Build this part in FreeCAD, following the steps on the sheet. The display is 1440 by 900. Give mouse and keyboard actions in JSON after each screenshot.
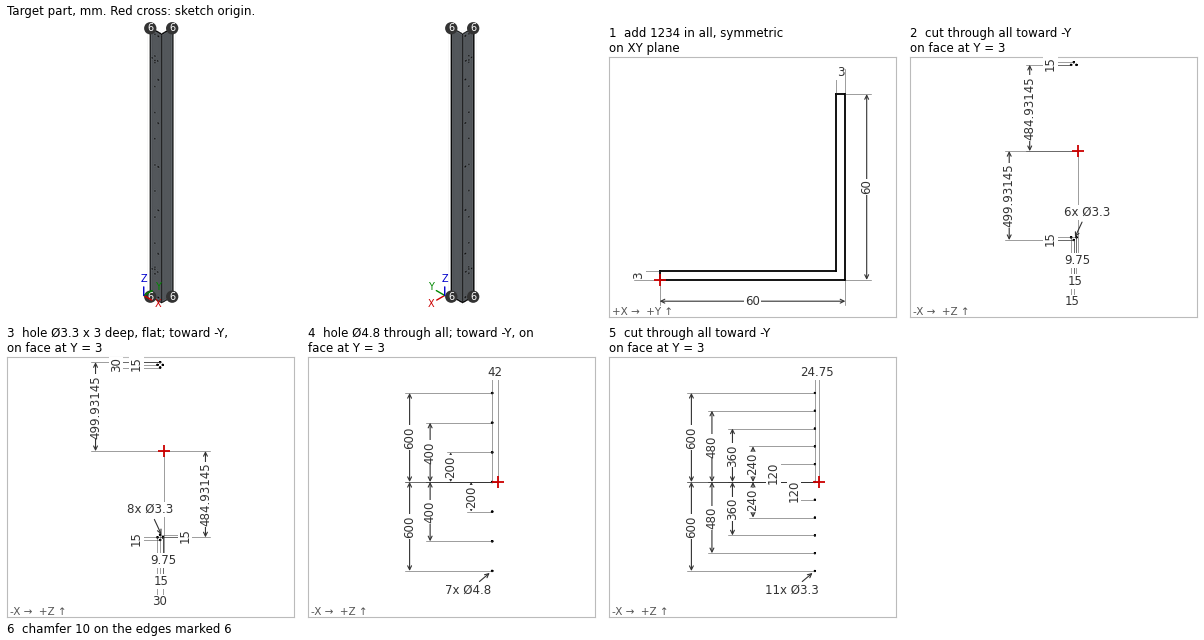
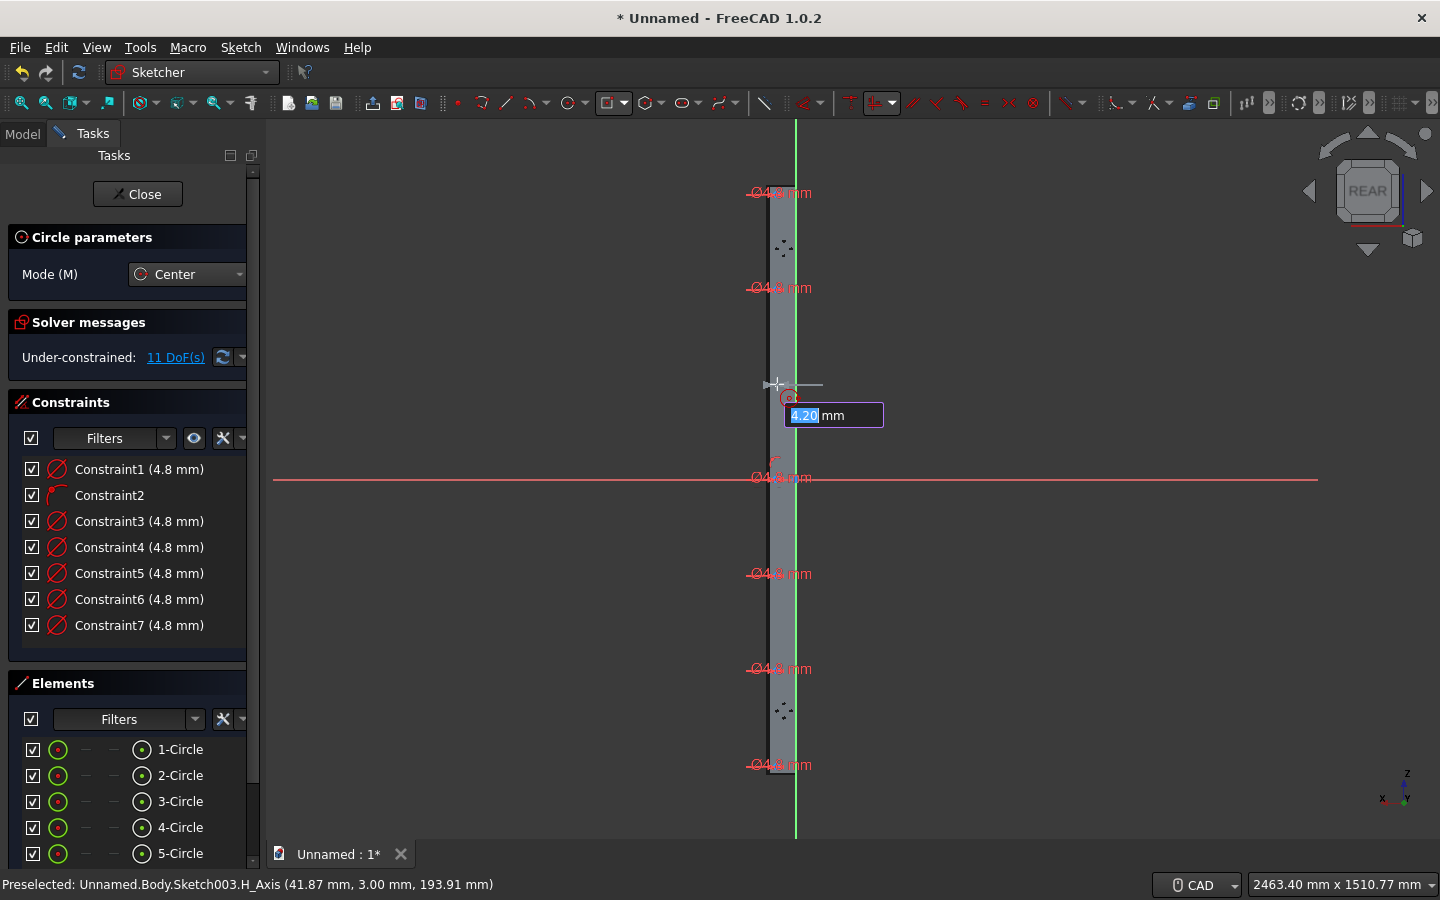
{"action": "type", "text": "4.8"}
{"action": "key", "text": "Return"}
{"action": "key", "text": "Escape"}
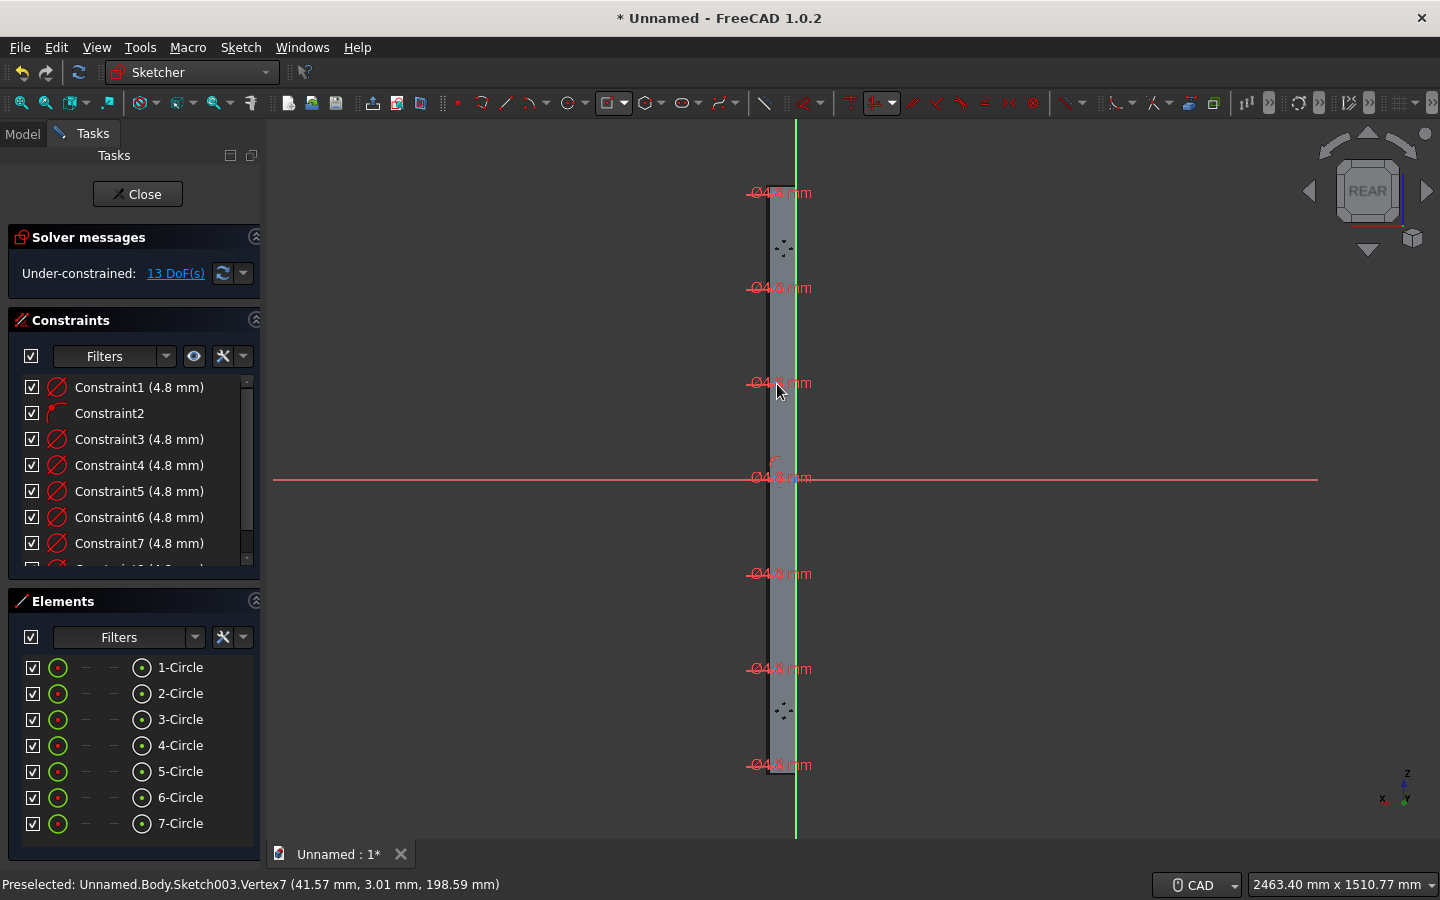
{"action": "left_click", "coordinate": [776, 480]}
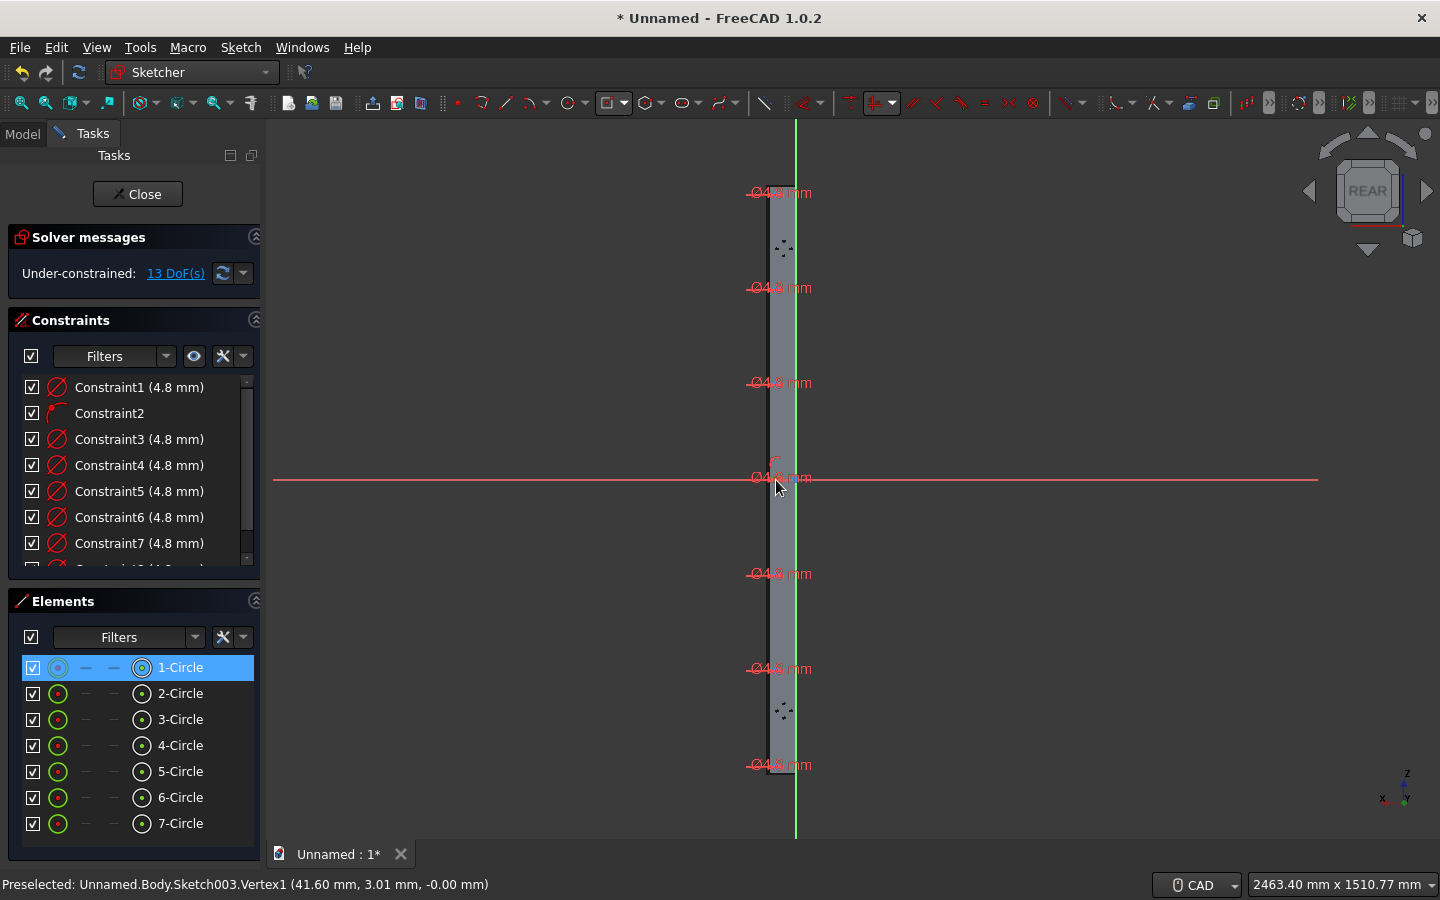
{"action": "left_click", "coordinate": [776, 576]}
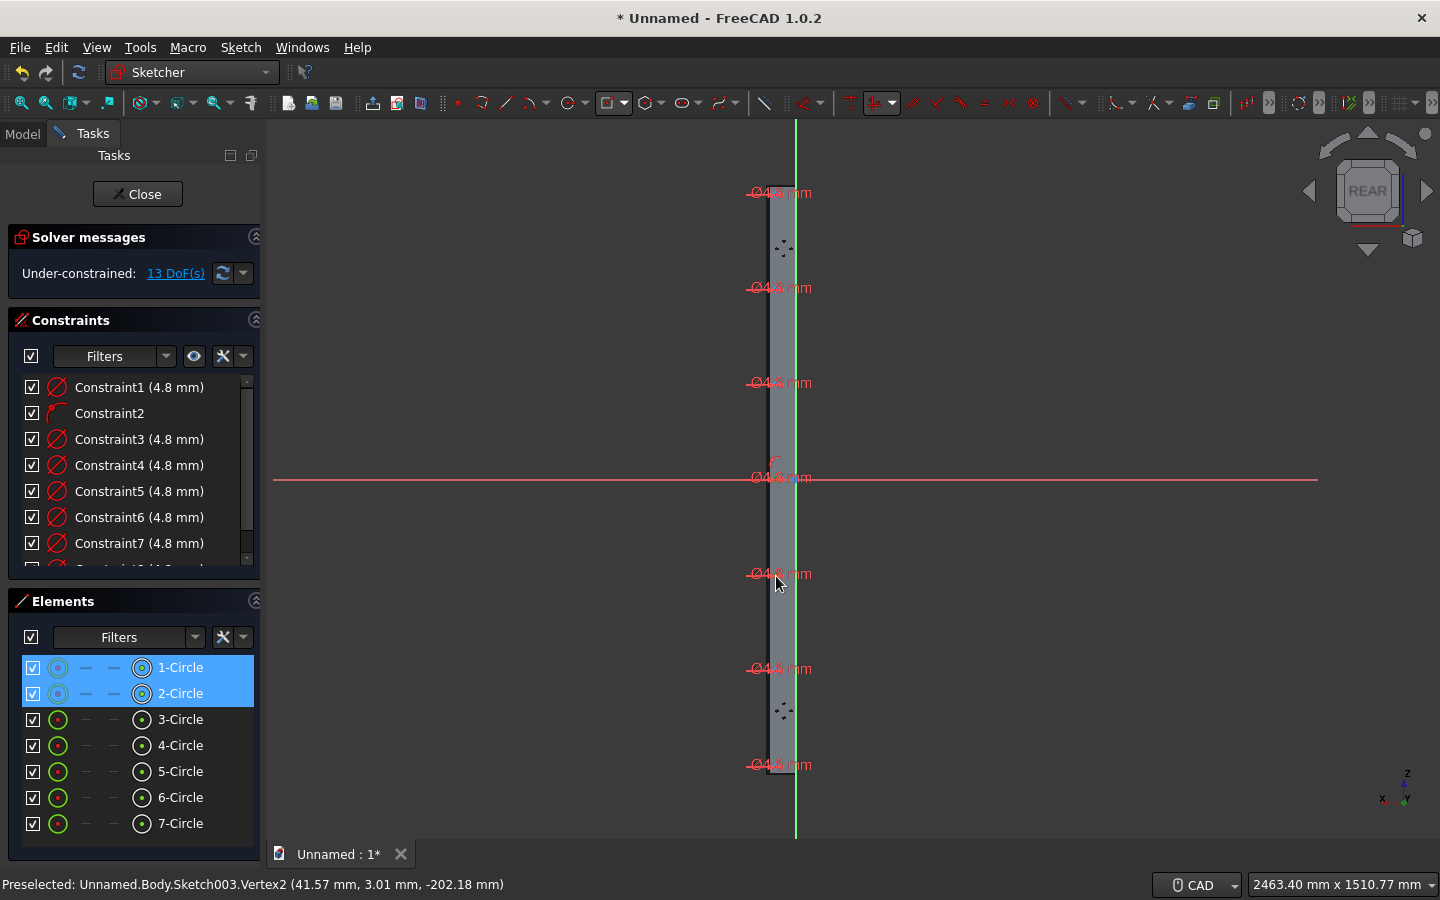
{"action": "left_click", "coordinate": [894, 104]}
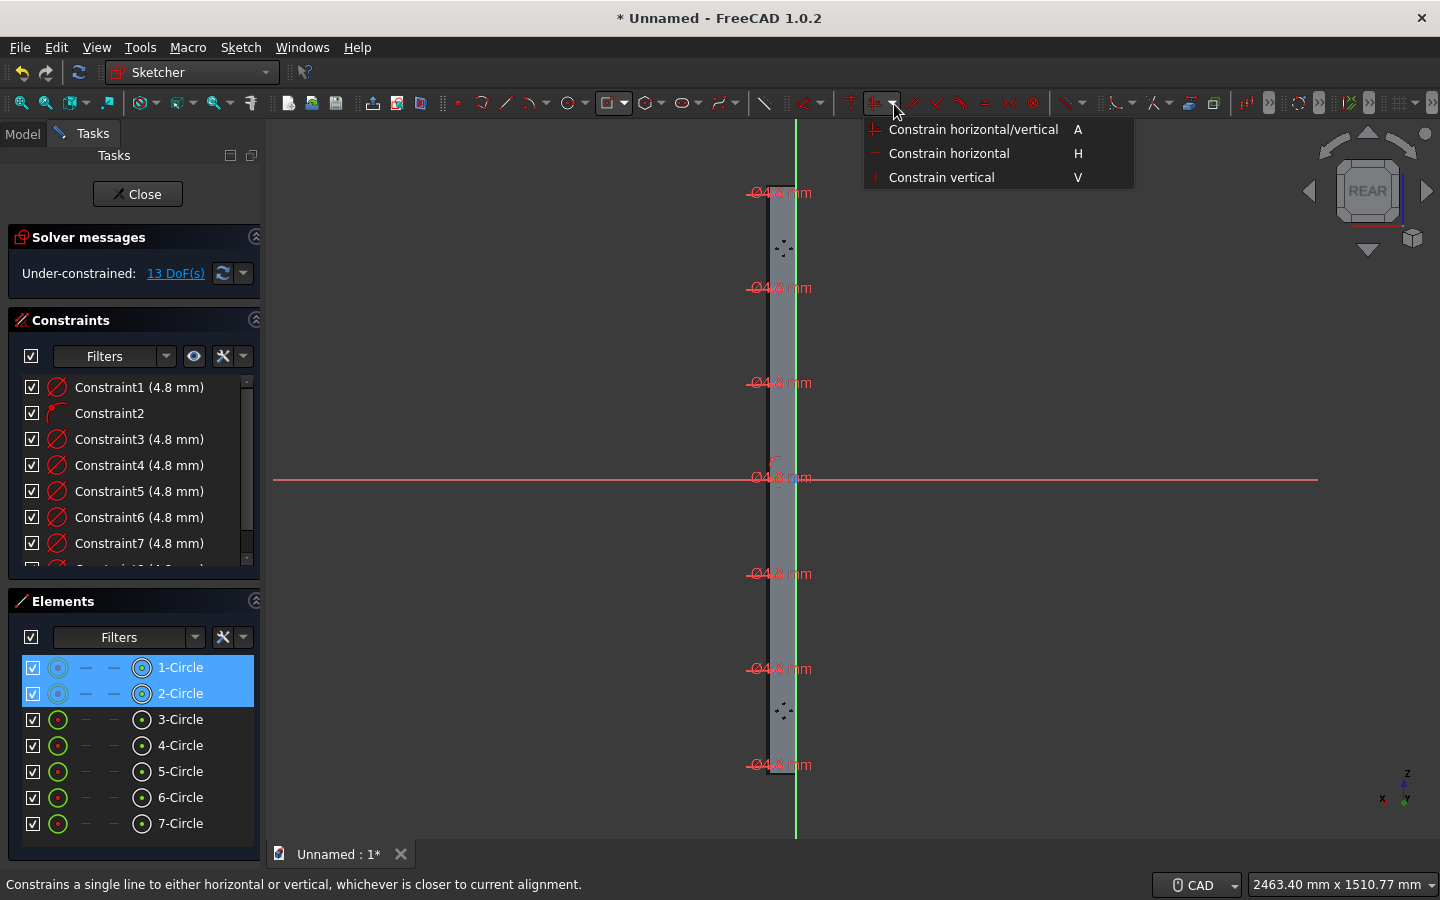
{"action": "left_click", "coordinate": [999, 177]}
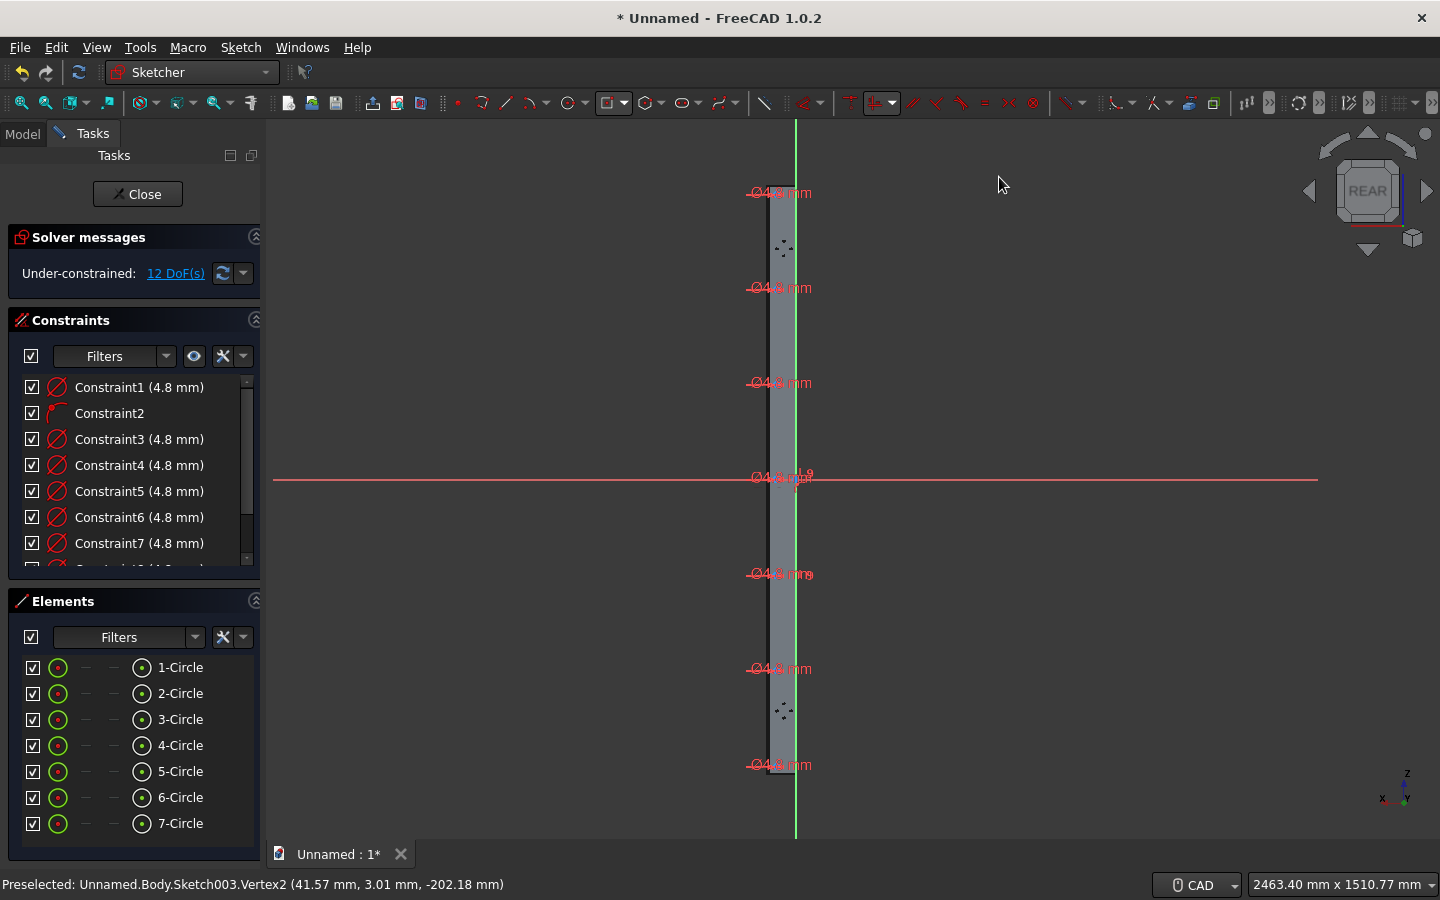
{"action": "left_click", "coordinate": [776, 576]}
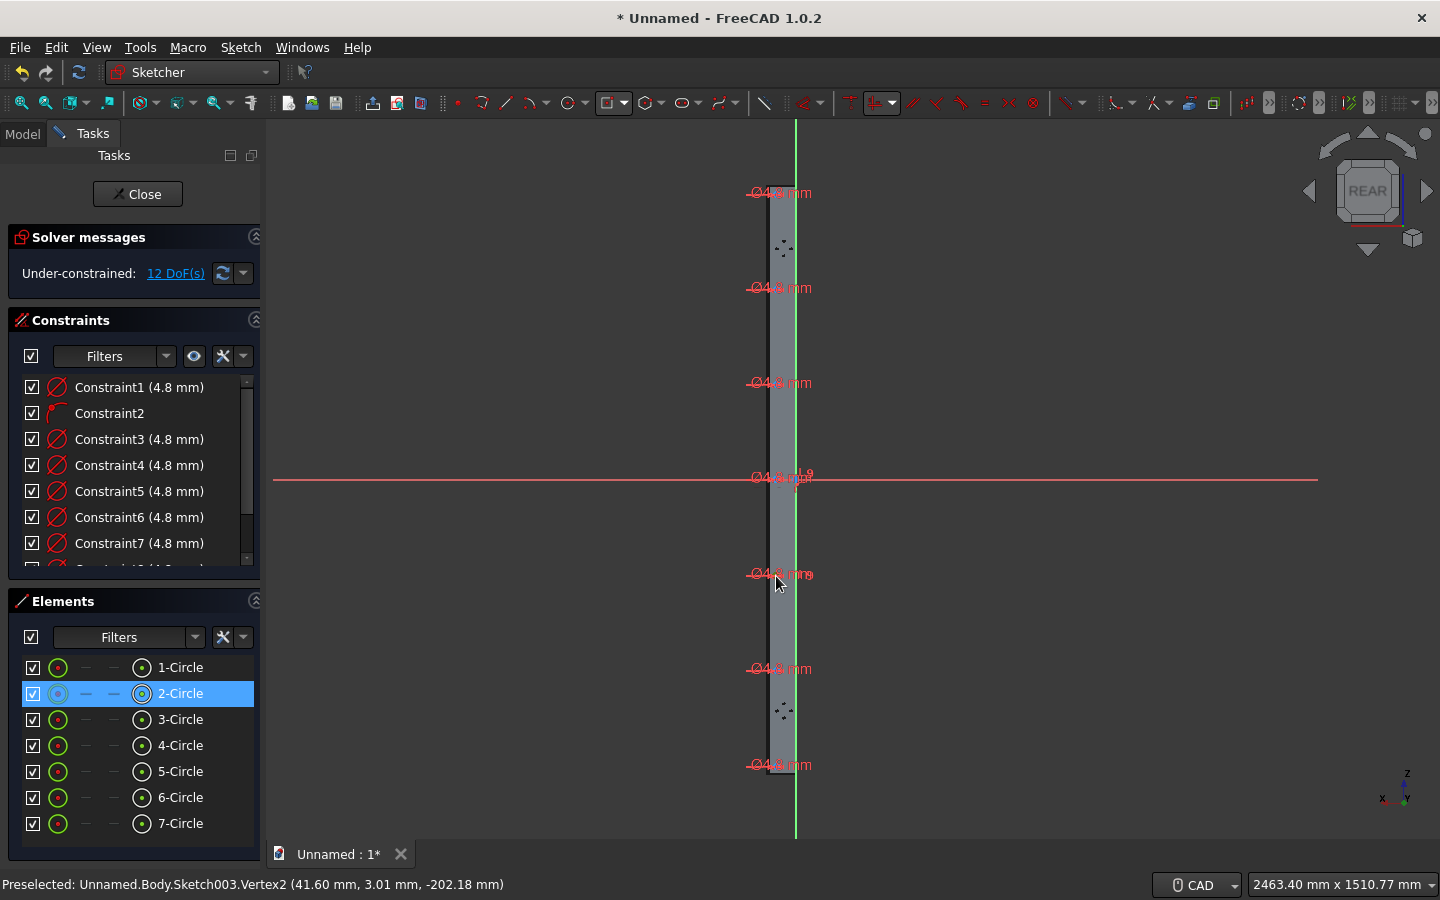
{"action": "left_click", "coordinate": [776, 671]}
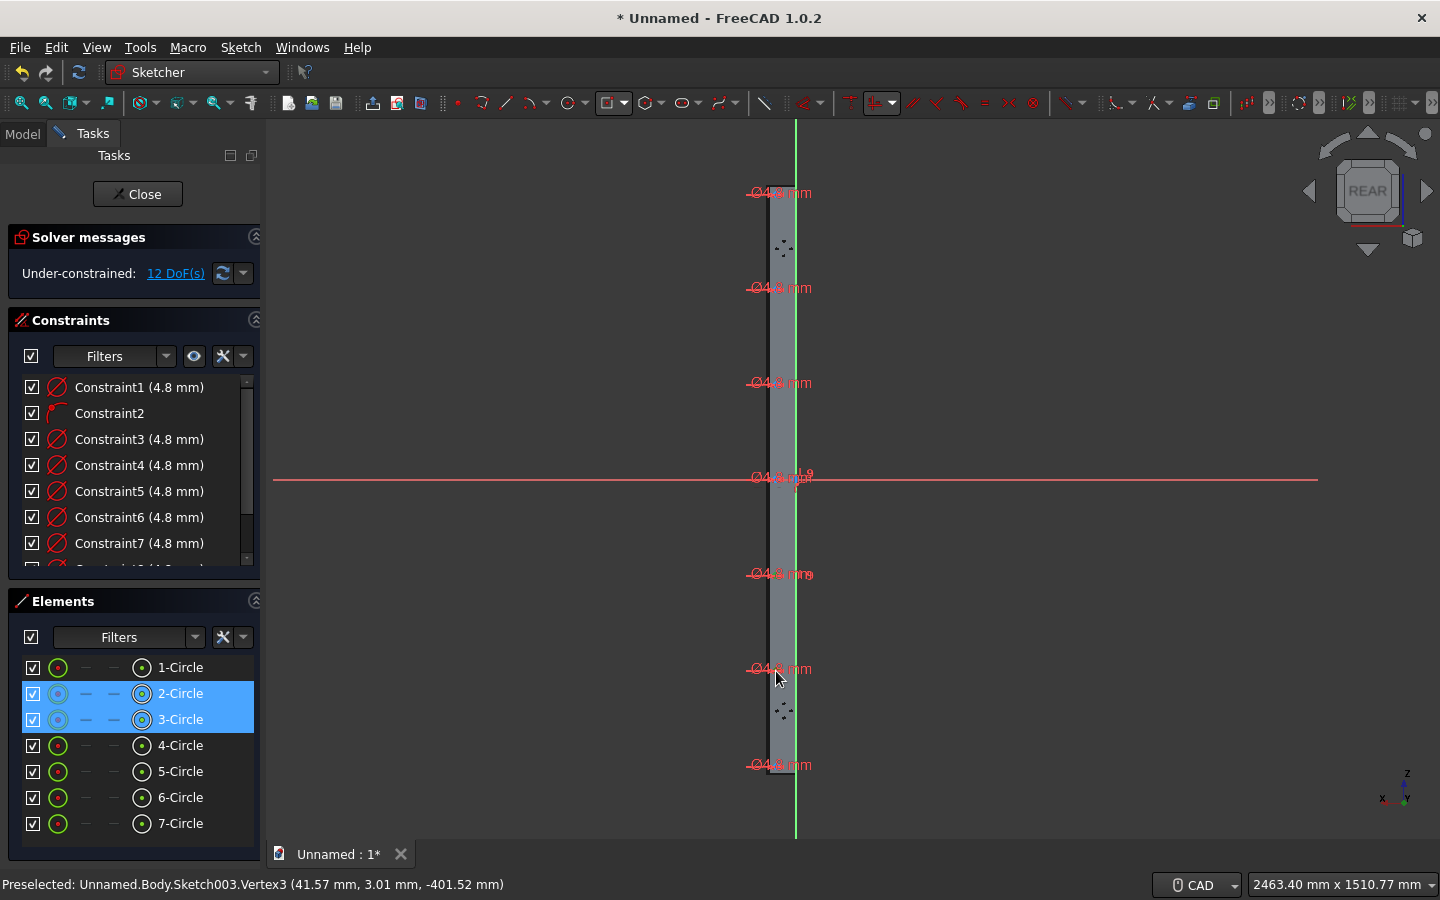
{"action": "left_click", "coordinate": [894, 104]}